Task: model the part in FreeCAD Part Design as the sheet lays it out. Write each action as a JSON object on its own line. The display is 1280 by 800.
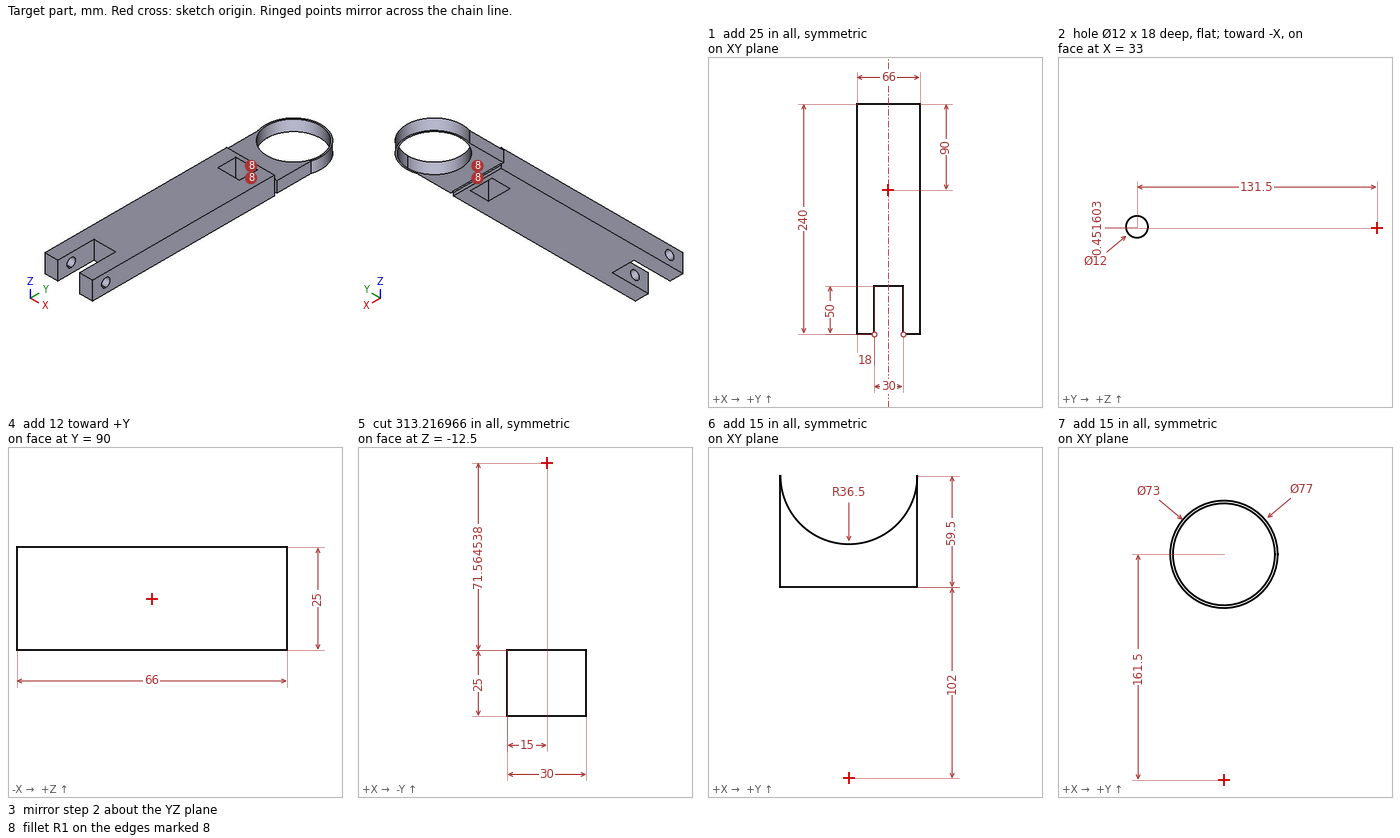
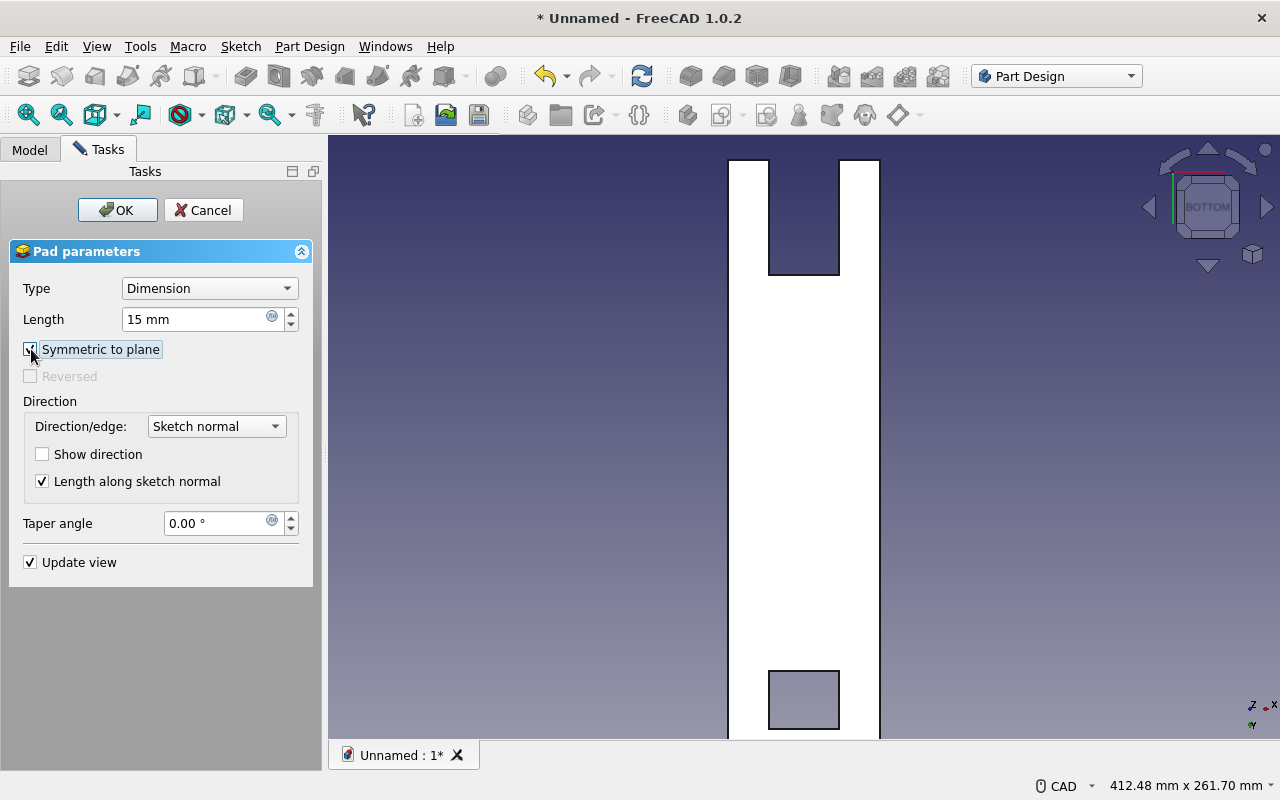
{"action": "left_click", "coordinate": [118, 210]}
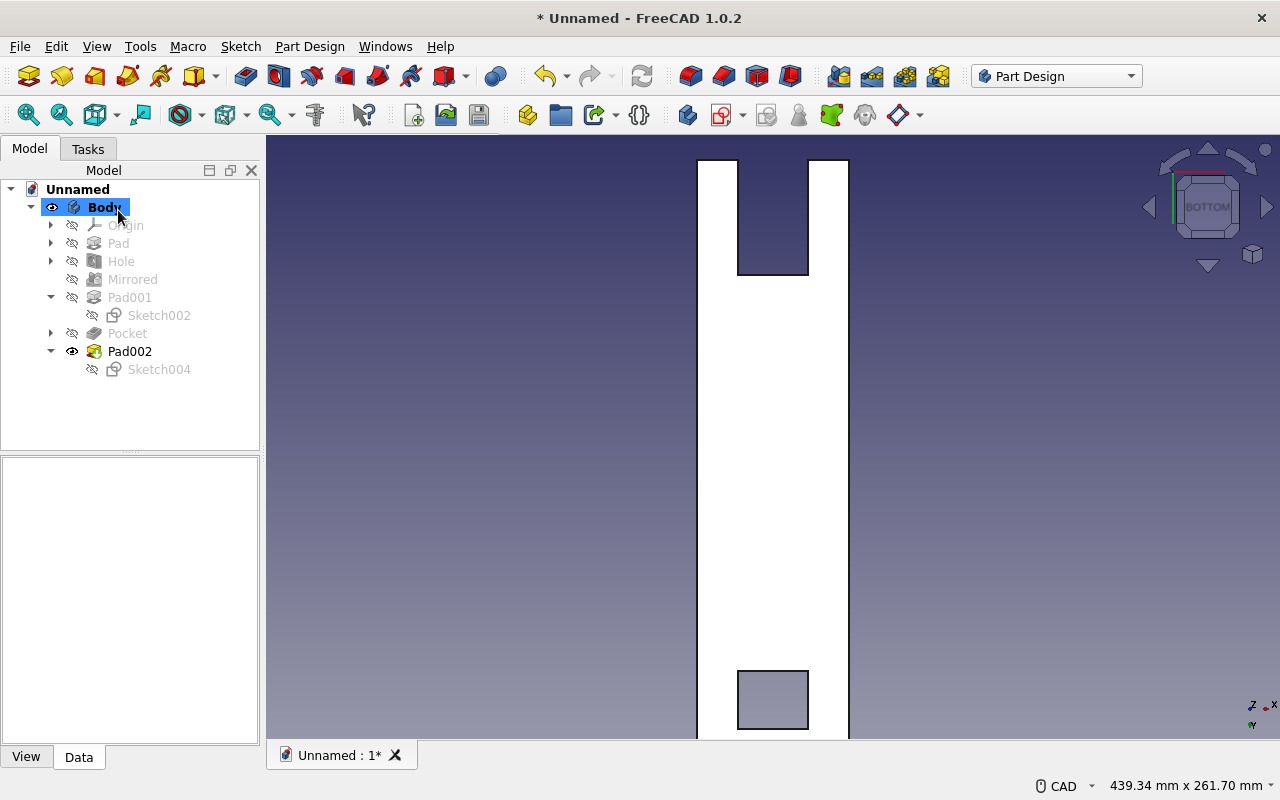
{"action": "left_click", "coordinate": [29, 116]}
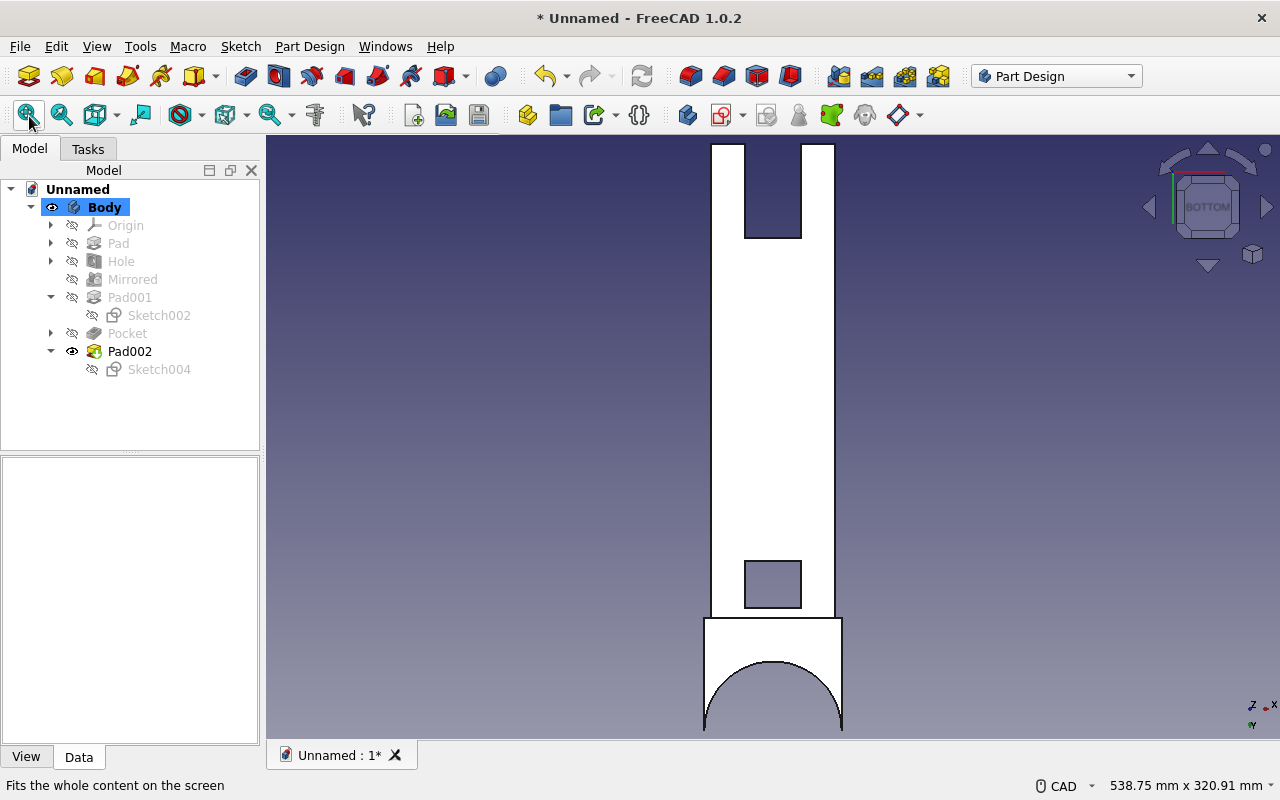
{"action": "left_click", "coordinate": [720, 116]}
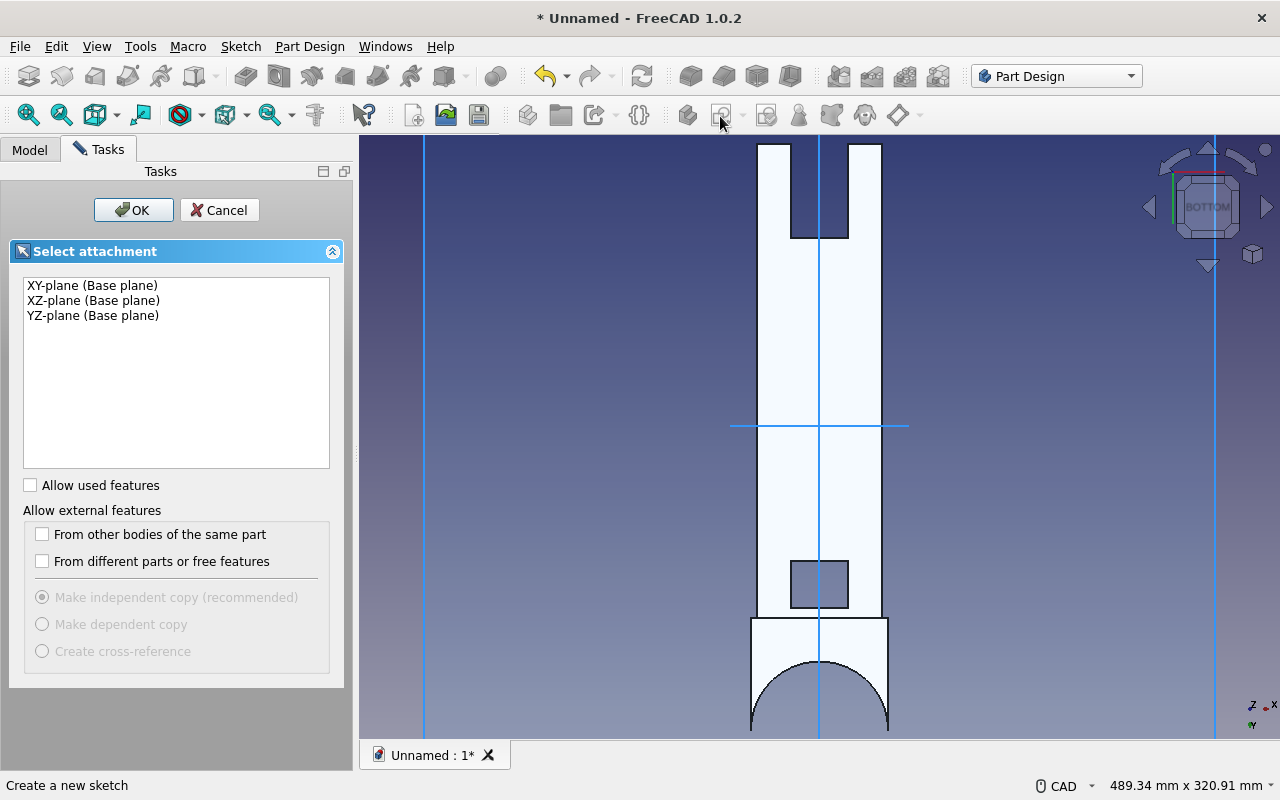
{"action": "left_click", "coordinate": [84, 286]}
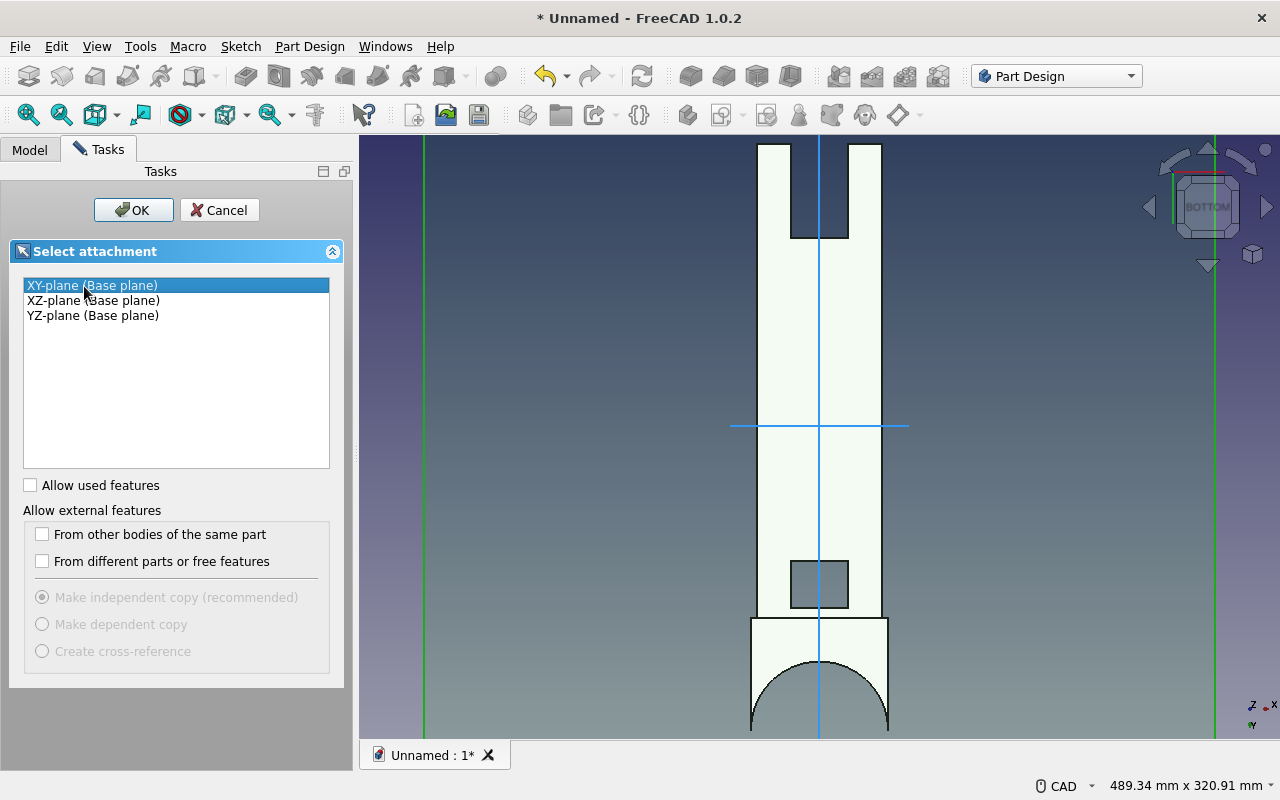
{"action": "left_click", "coordinate": [134, 210]}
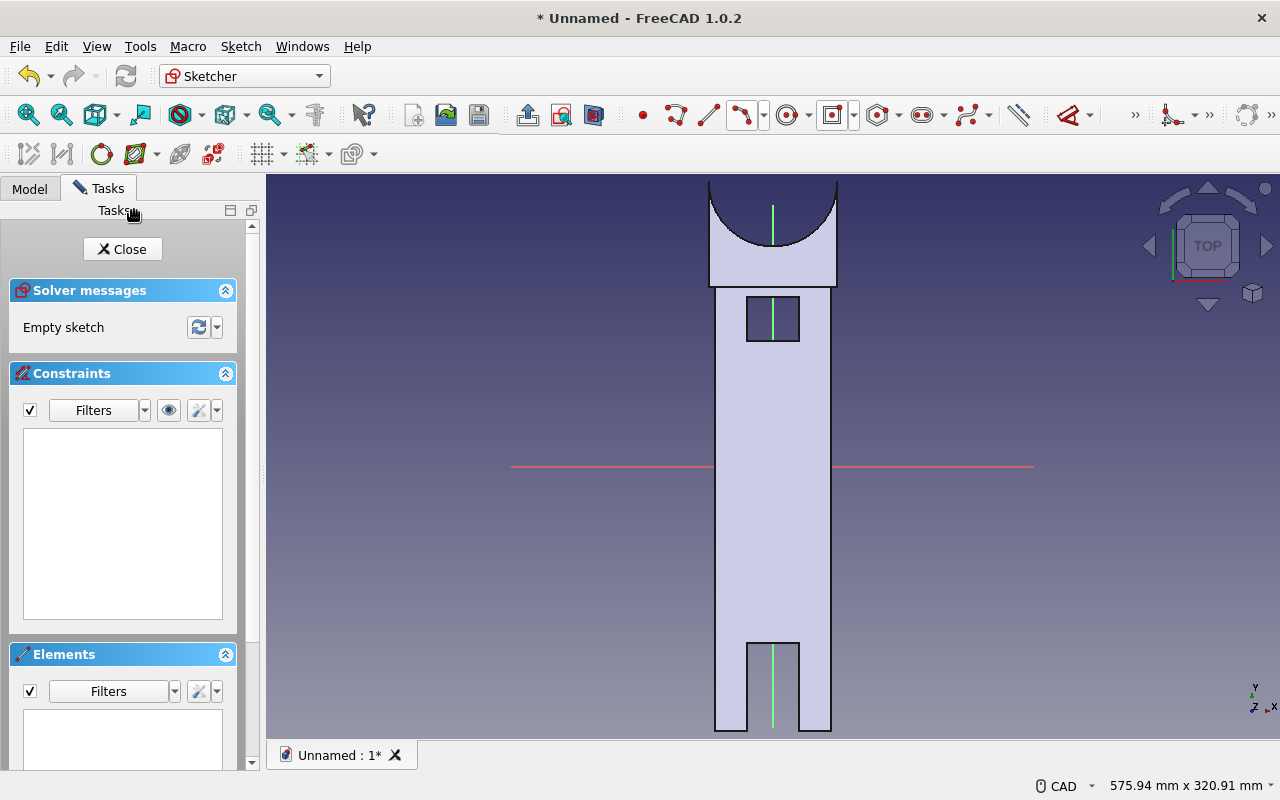
{"action": "key", "text": "q s"}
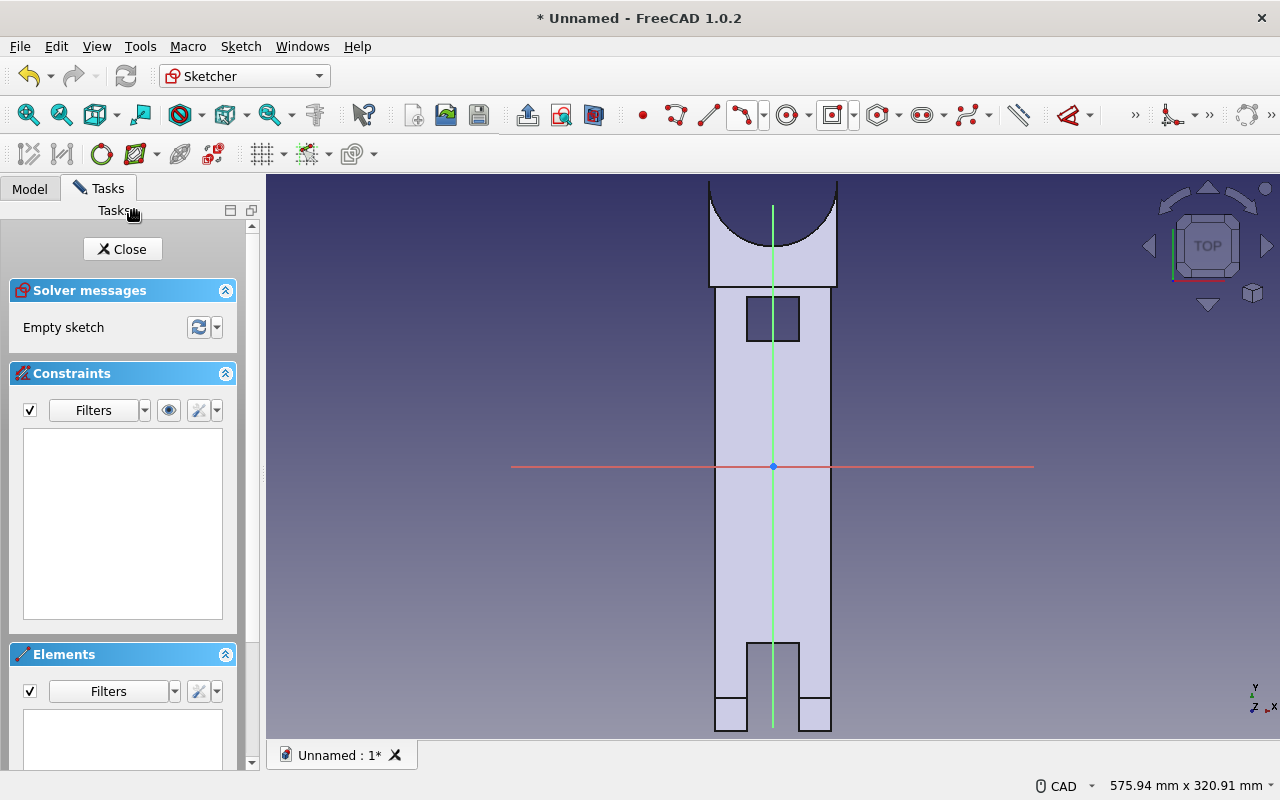
{"action": "scroll", "coordinate": [704, 456], "scroll_direction": "down", "scroll_amount": 5}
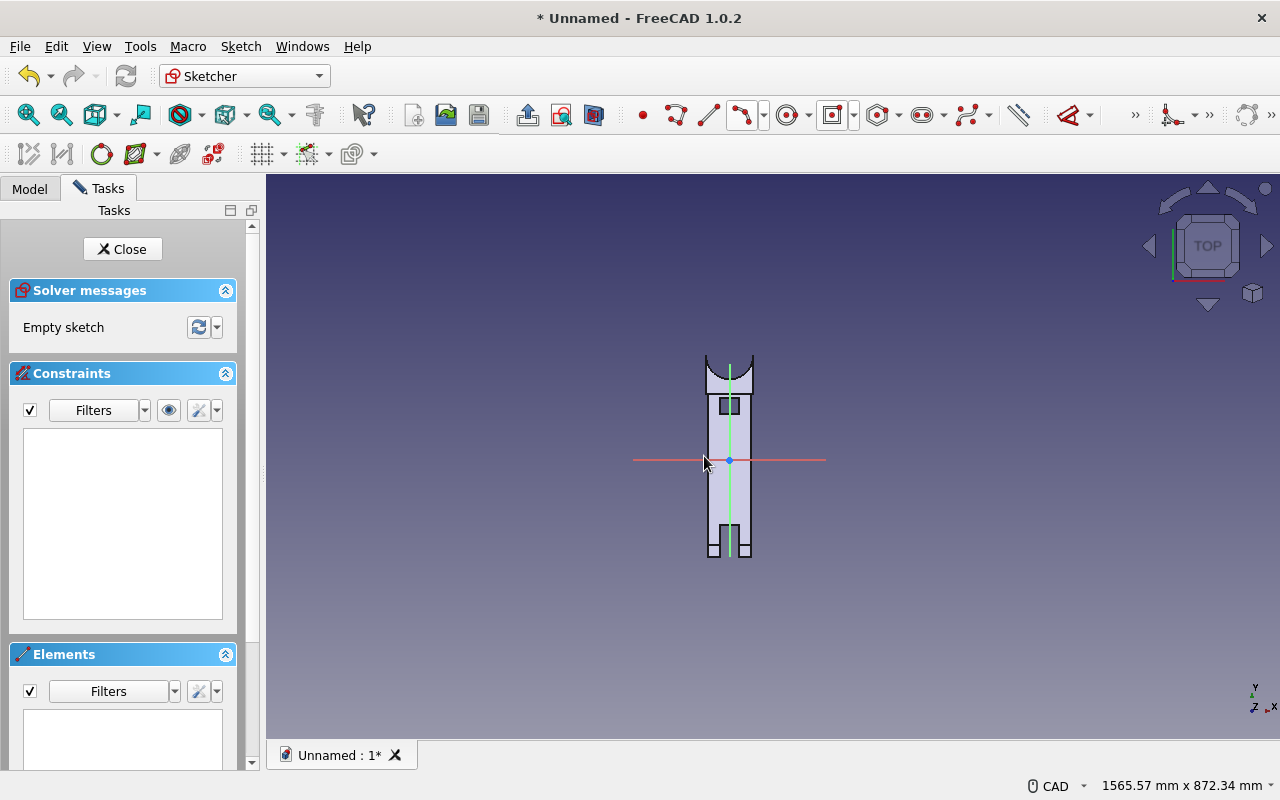
{"action": "scroll", "coordinate": [734, 340], "scroll_direction": "up", "scroll_amount": 10}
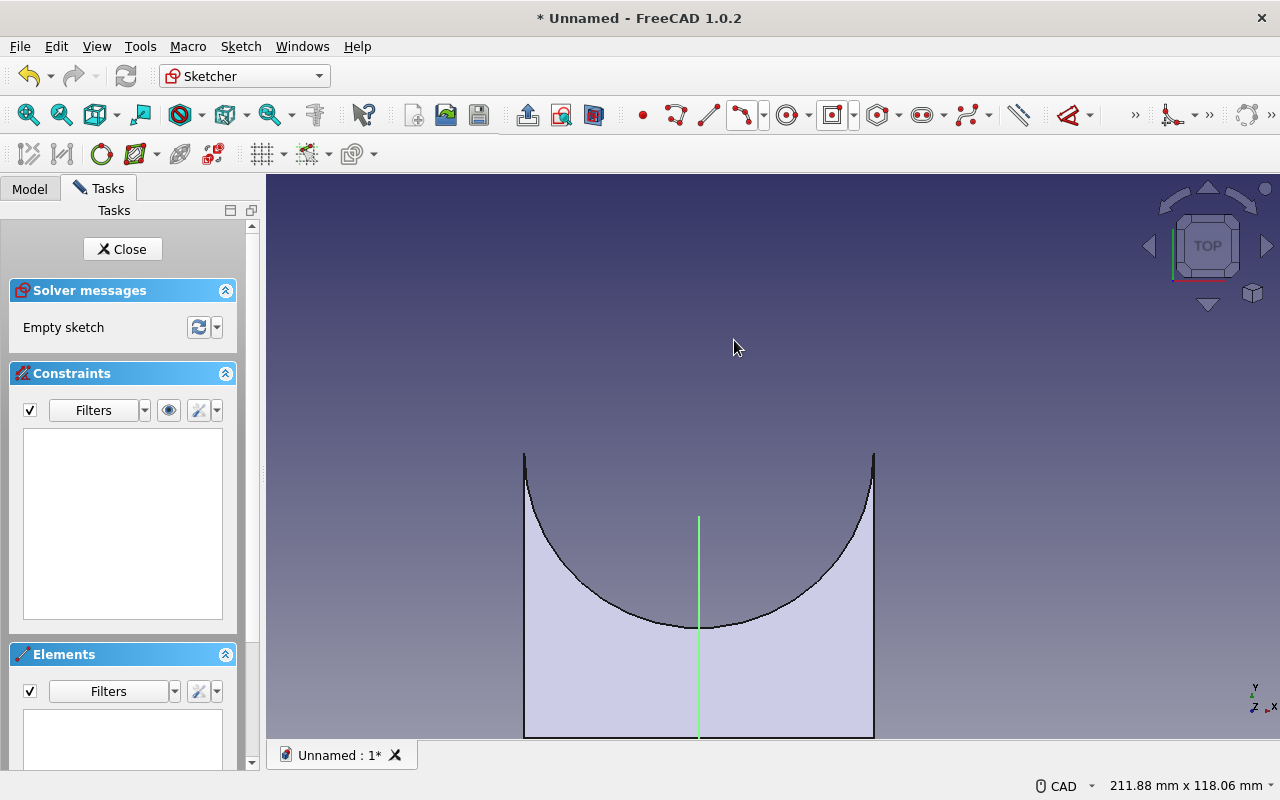
{"action": "key", "text": "g c"}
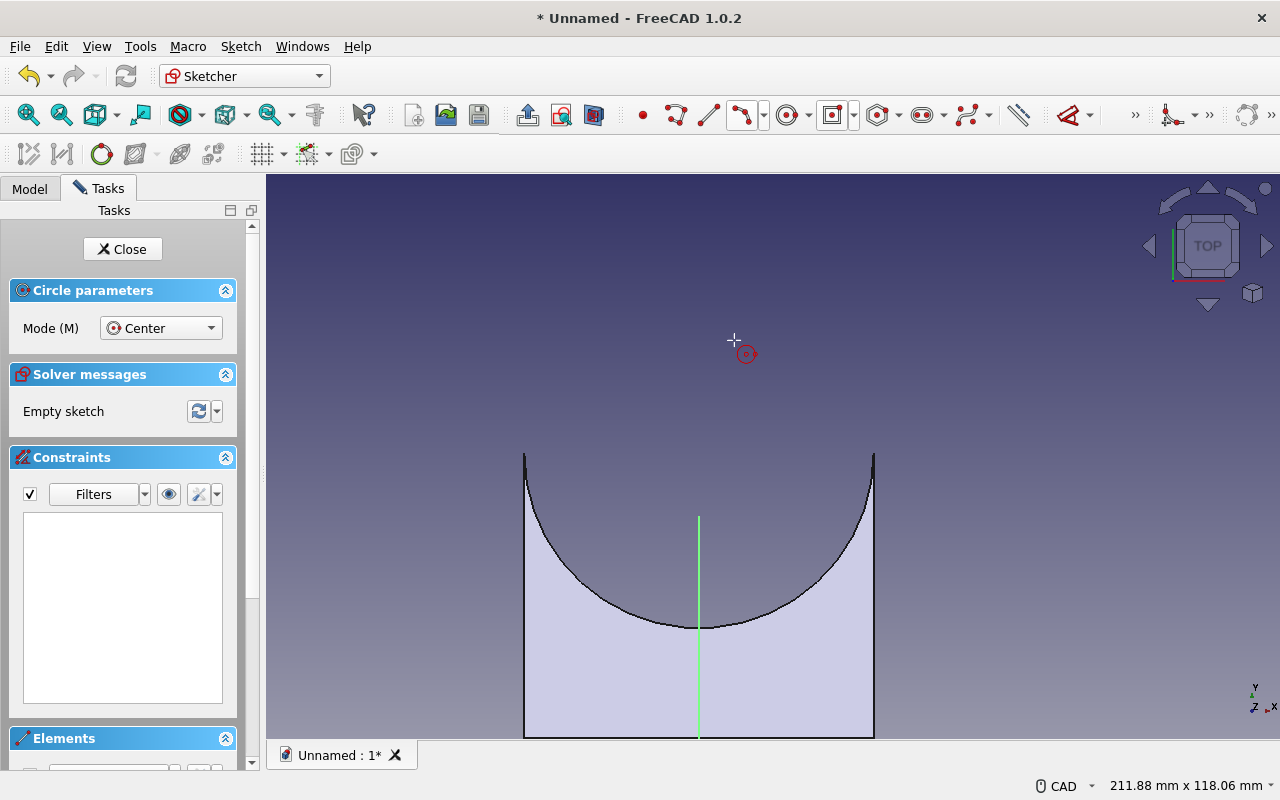
{"action": "left_click", "coordinate": [699, 454]}
{"action": "left_click", "coordinate": [829, 323]}